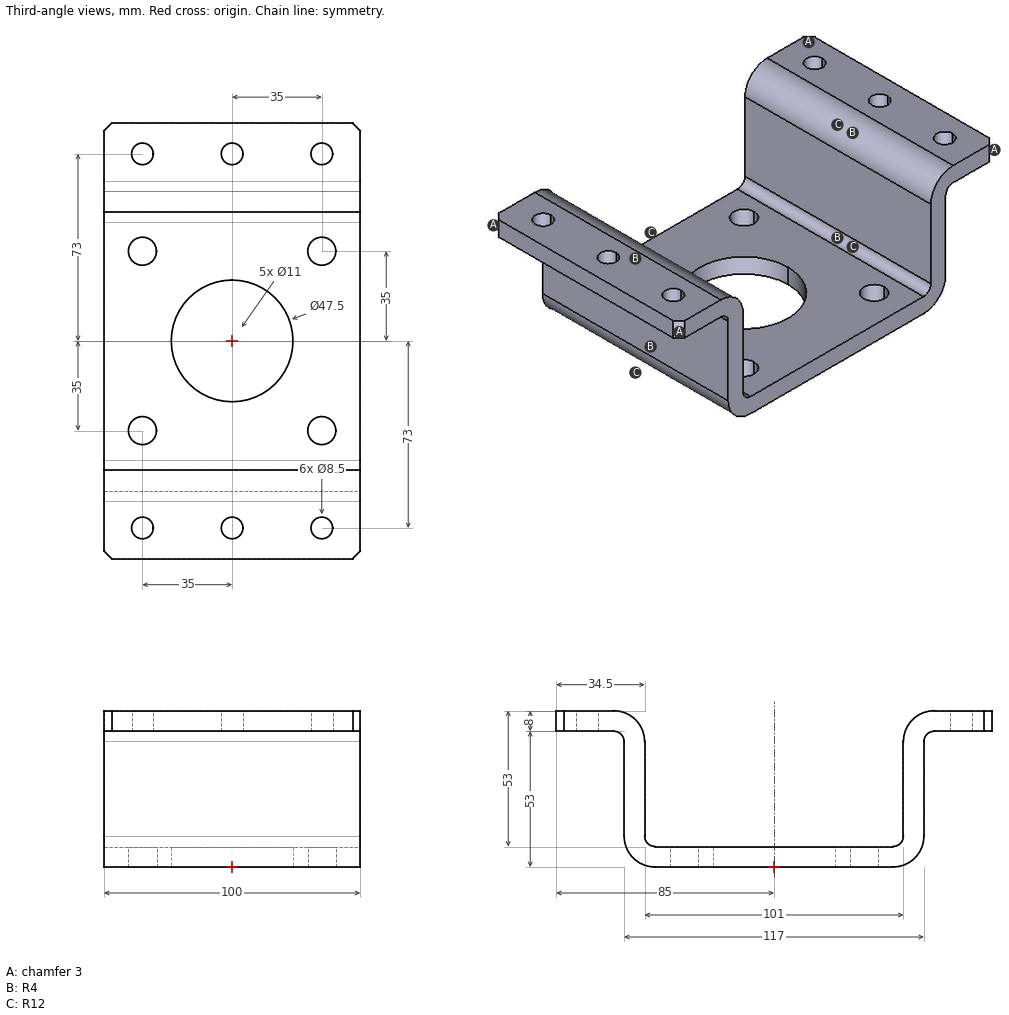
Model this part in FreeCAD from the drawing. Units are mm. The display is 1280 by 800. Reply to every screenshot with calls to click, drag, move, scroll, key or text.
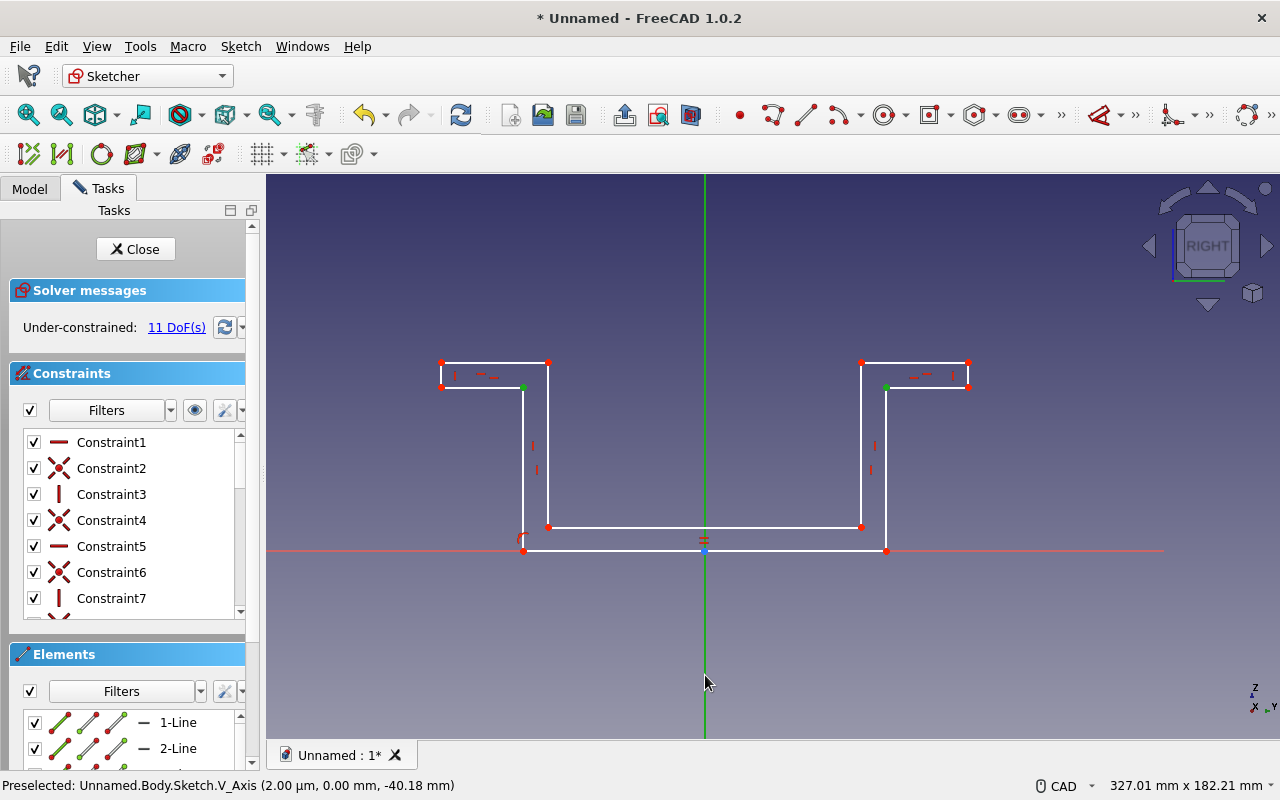
key(s)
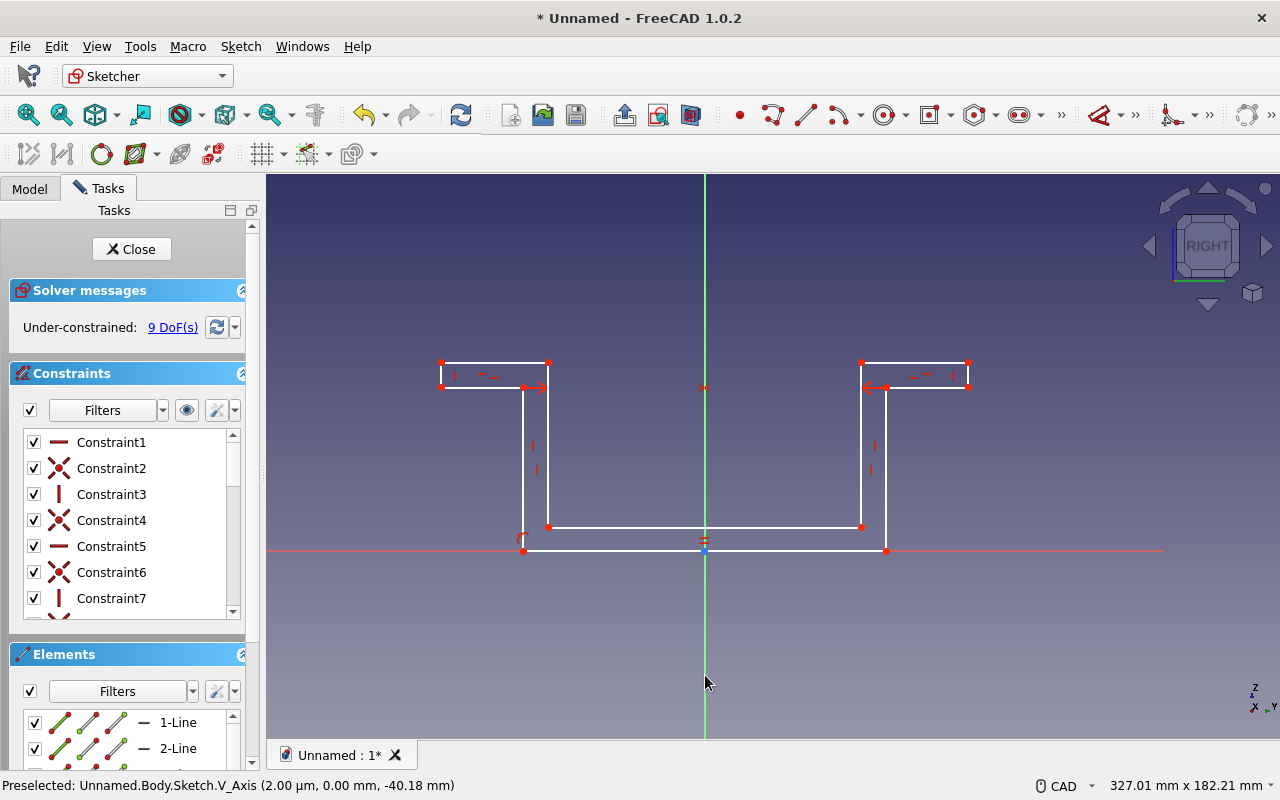
click(441, 363)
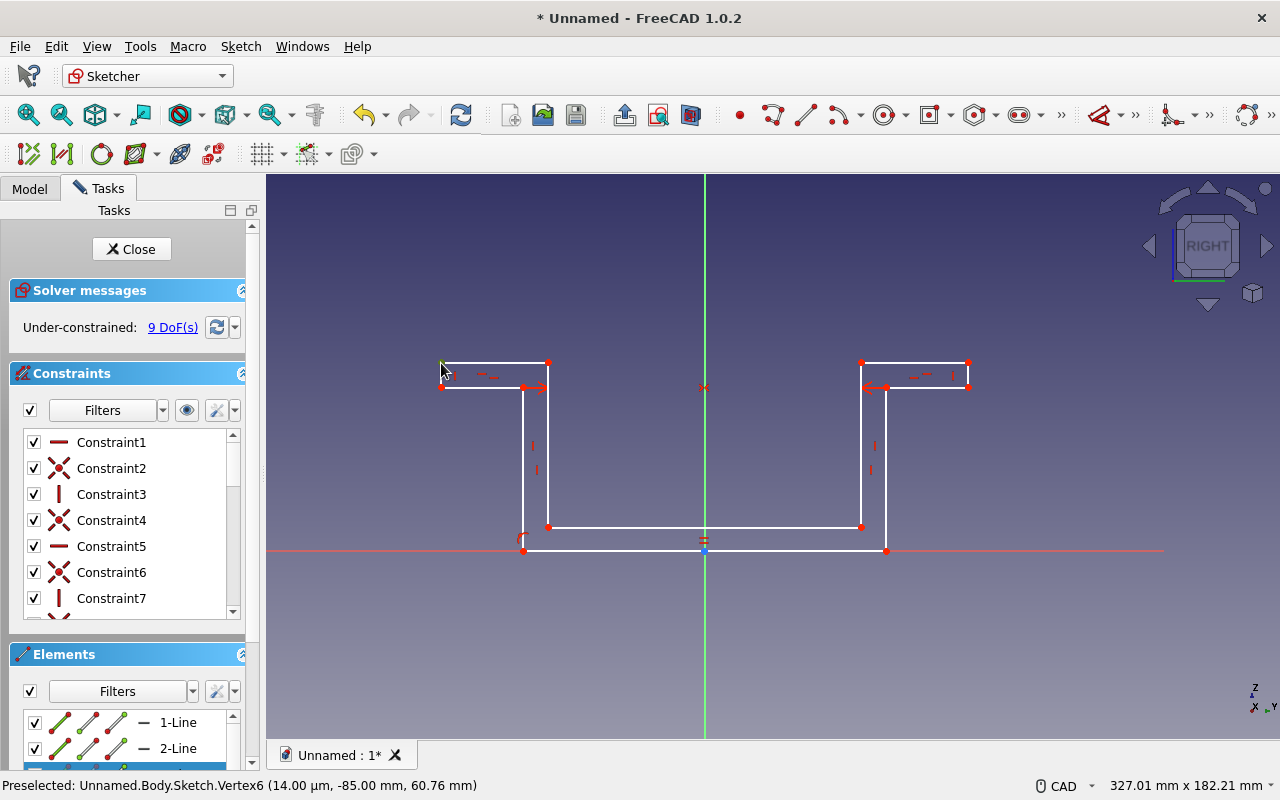
click(968, 363)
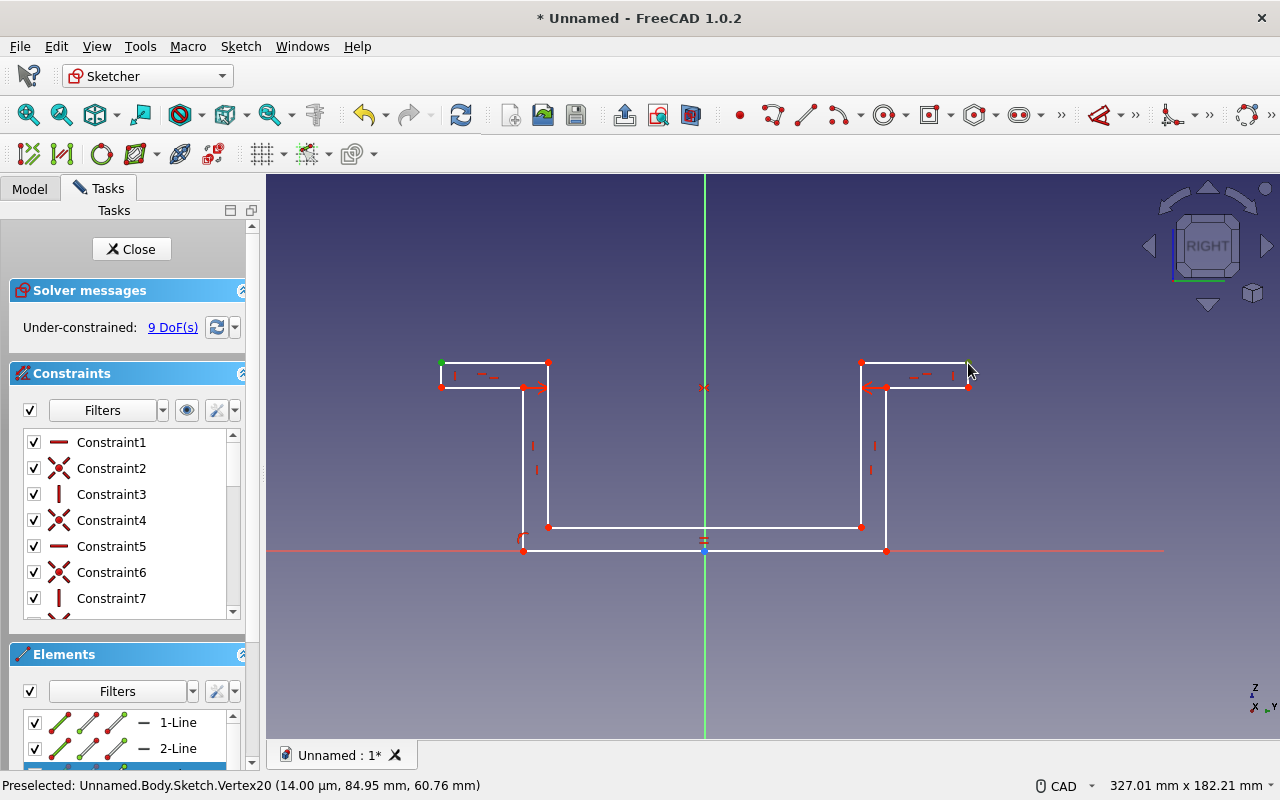
click(705, 675)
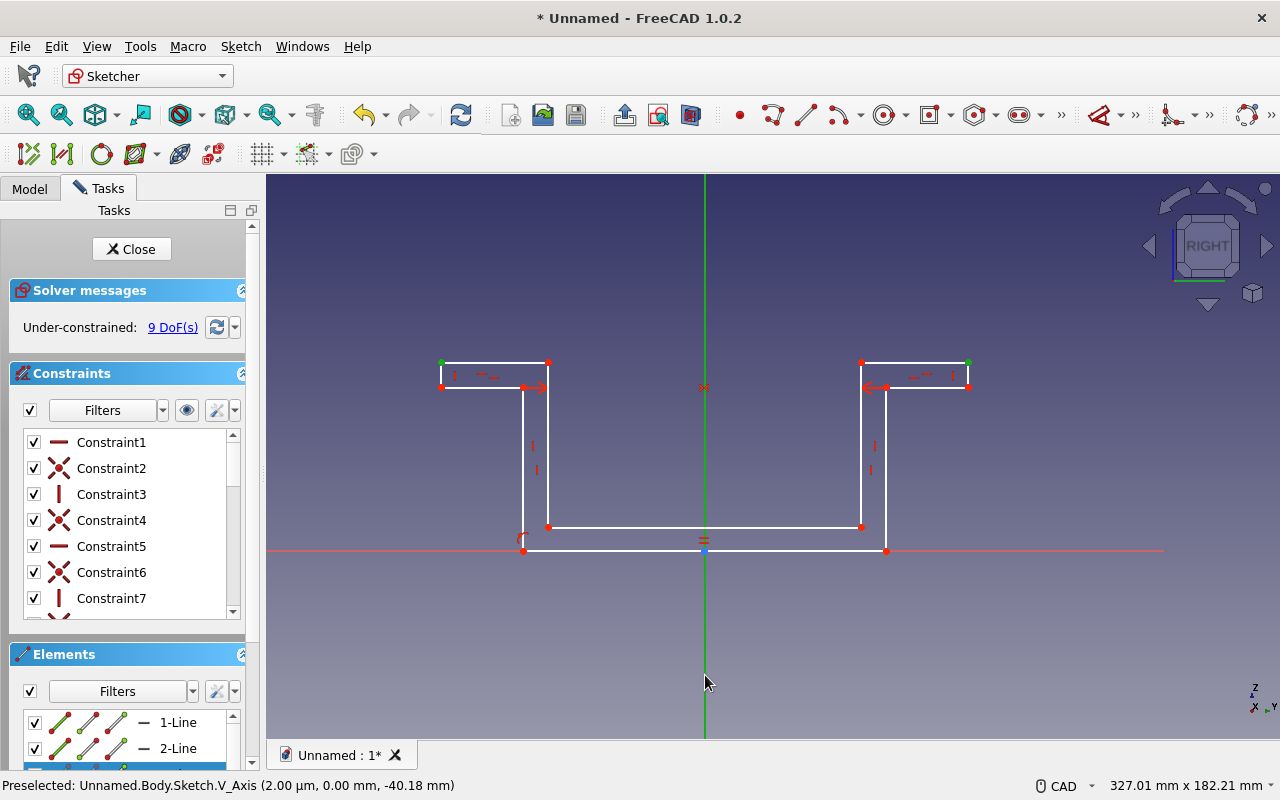
key(s)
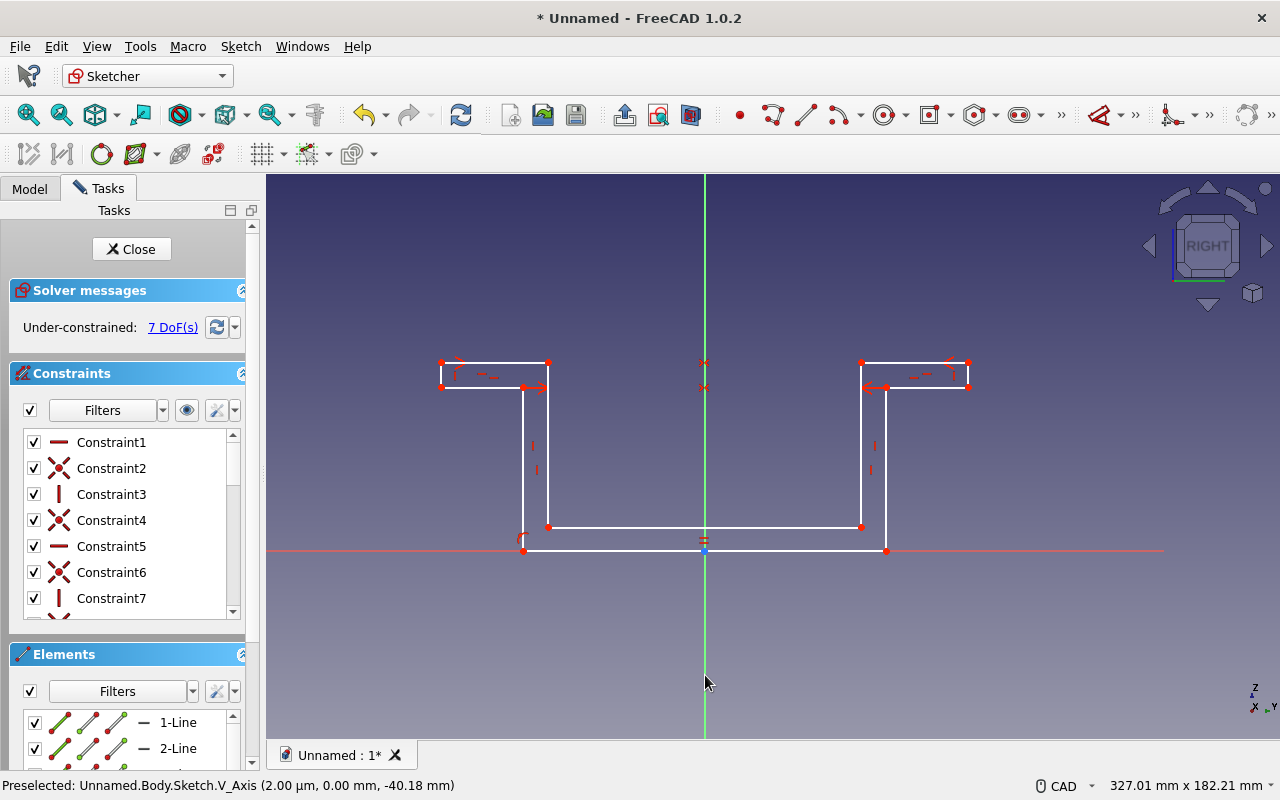
key(d)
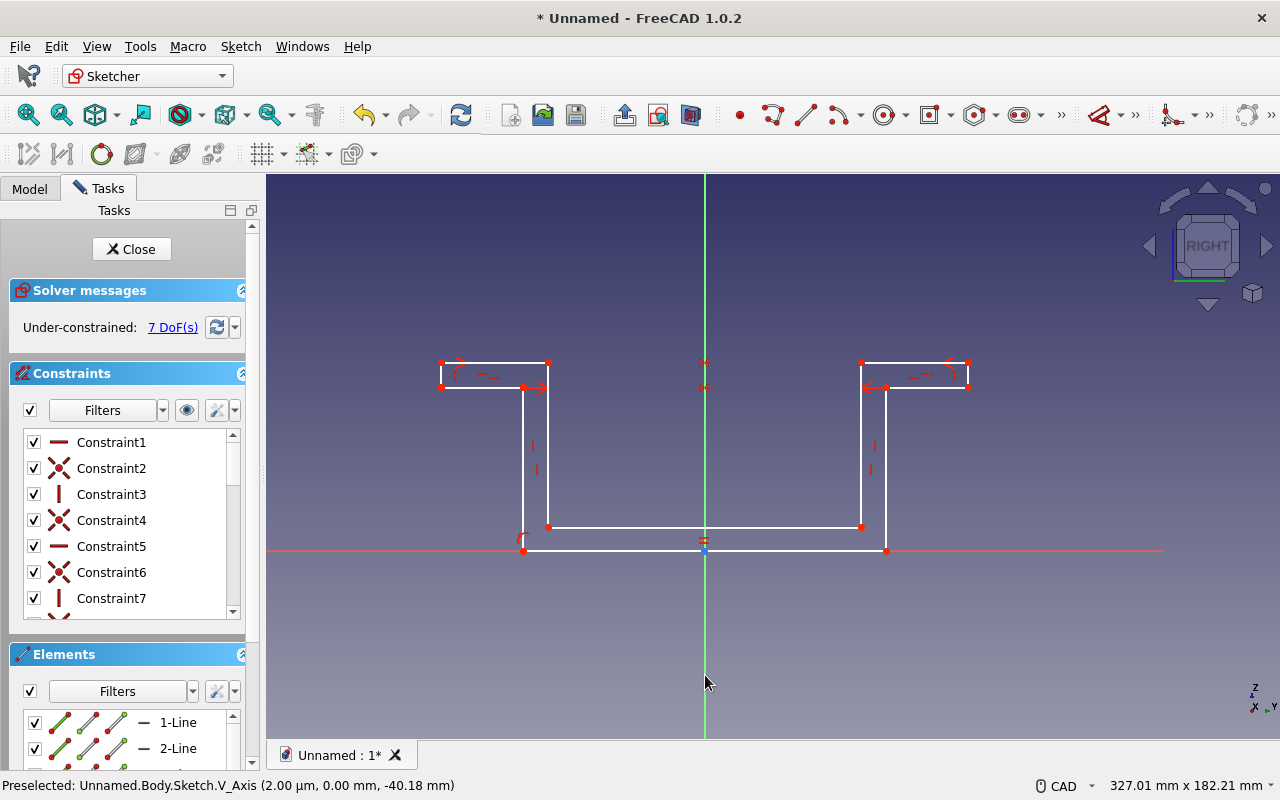
scroll(441, 373, up, 3)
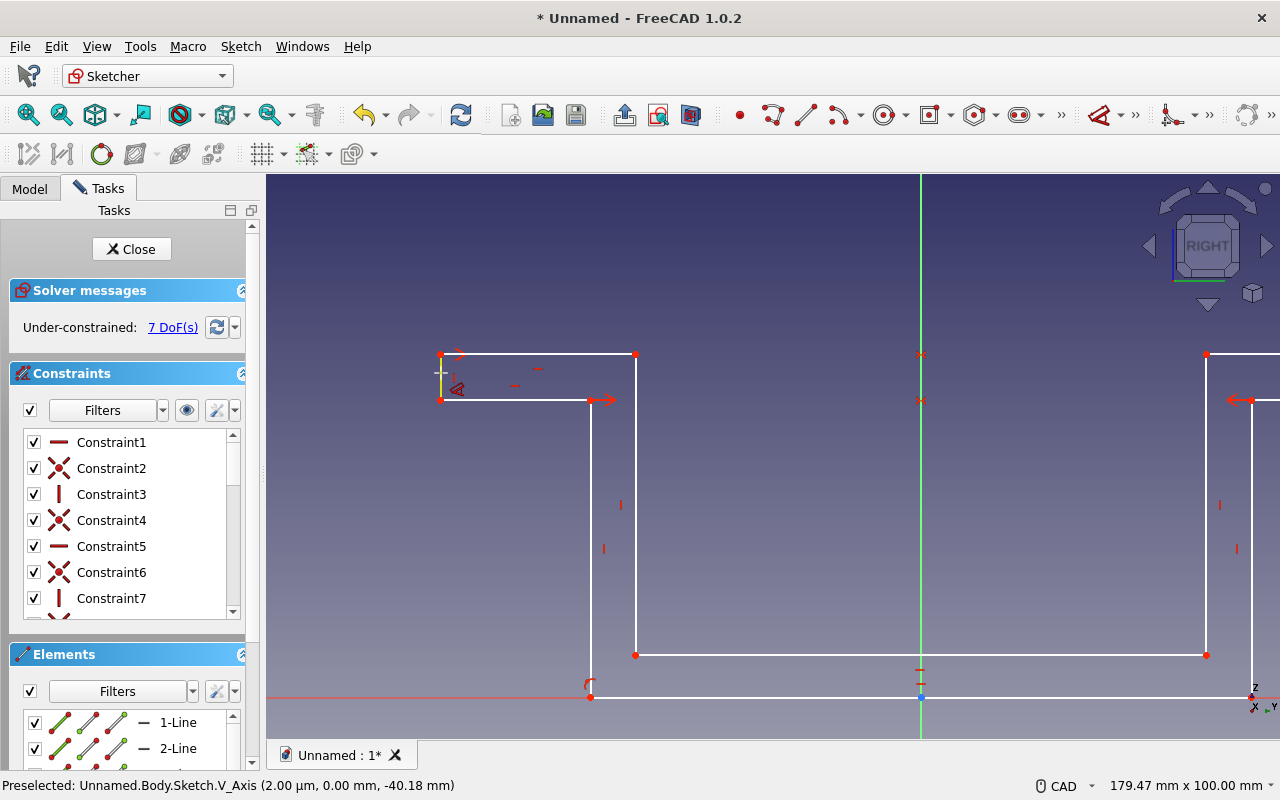
click(441, 373)
click(407, 377)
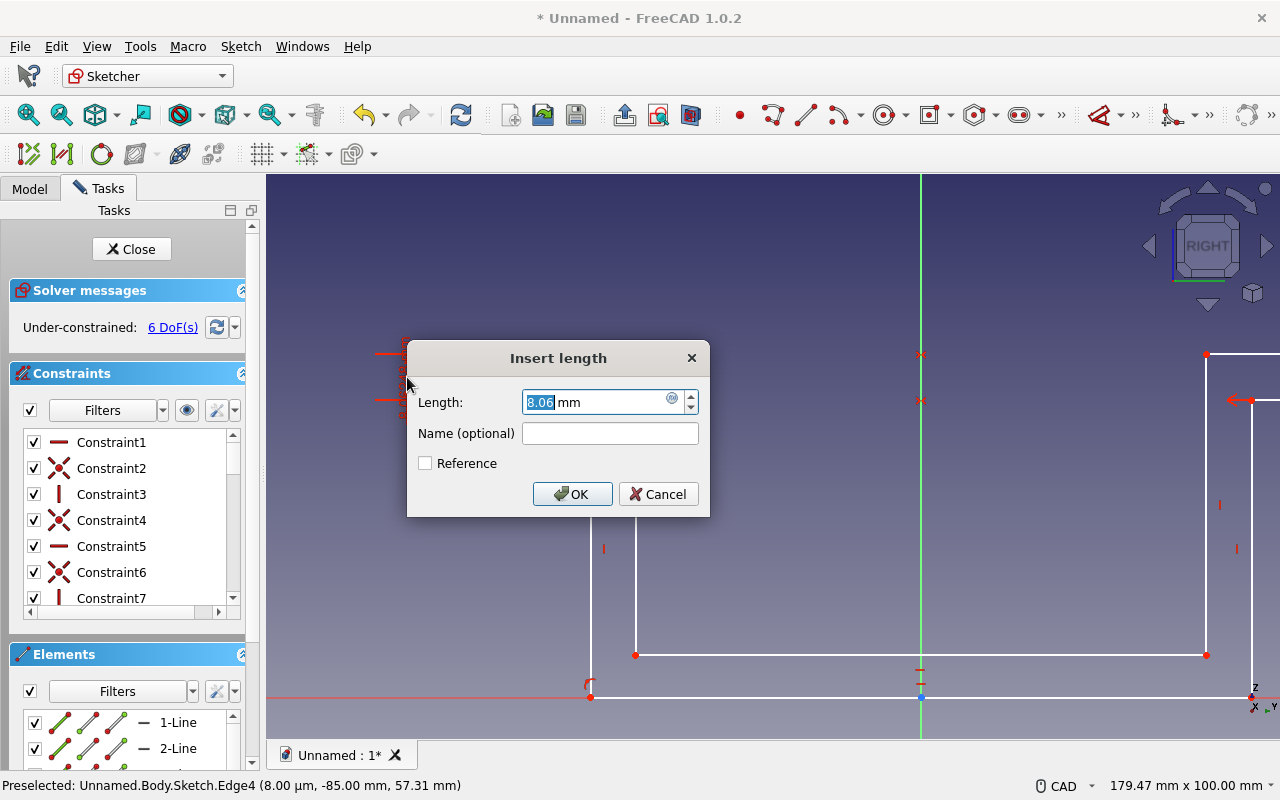
text(8)
key(Return)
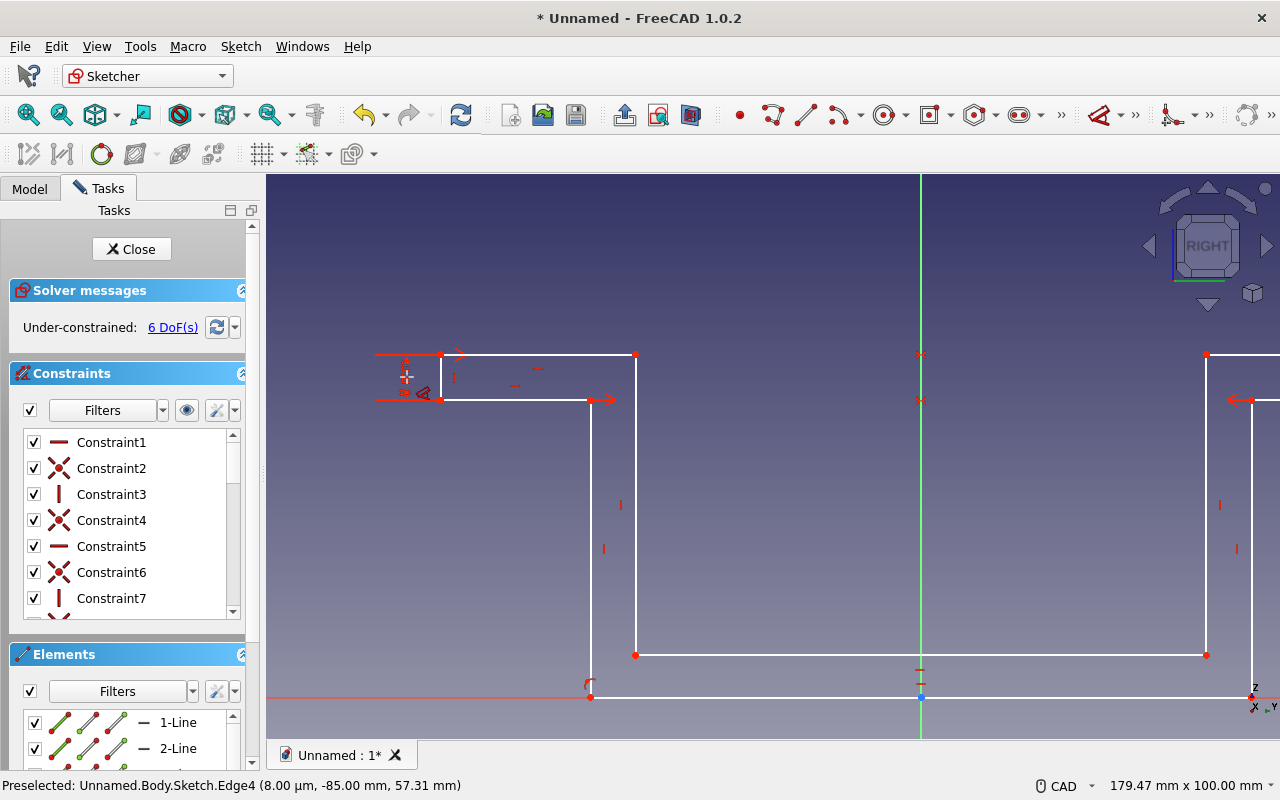
click(636, 565)
click(670, 505)